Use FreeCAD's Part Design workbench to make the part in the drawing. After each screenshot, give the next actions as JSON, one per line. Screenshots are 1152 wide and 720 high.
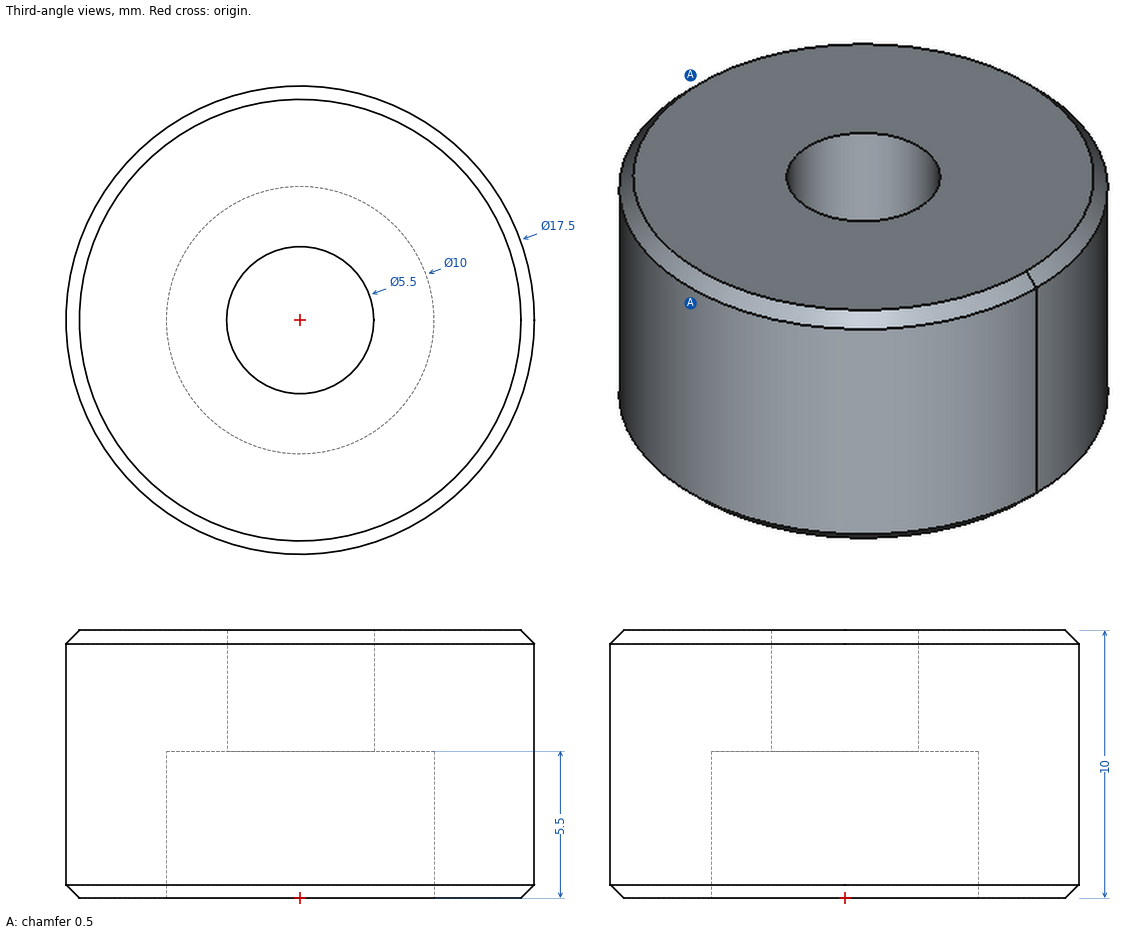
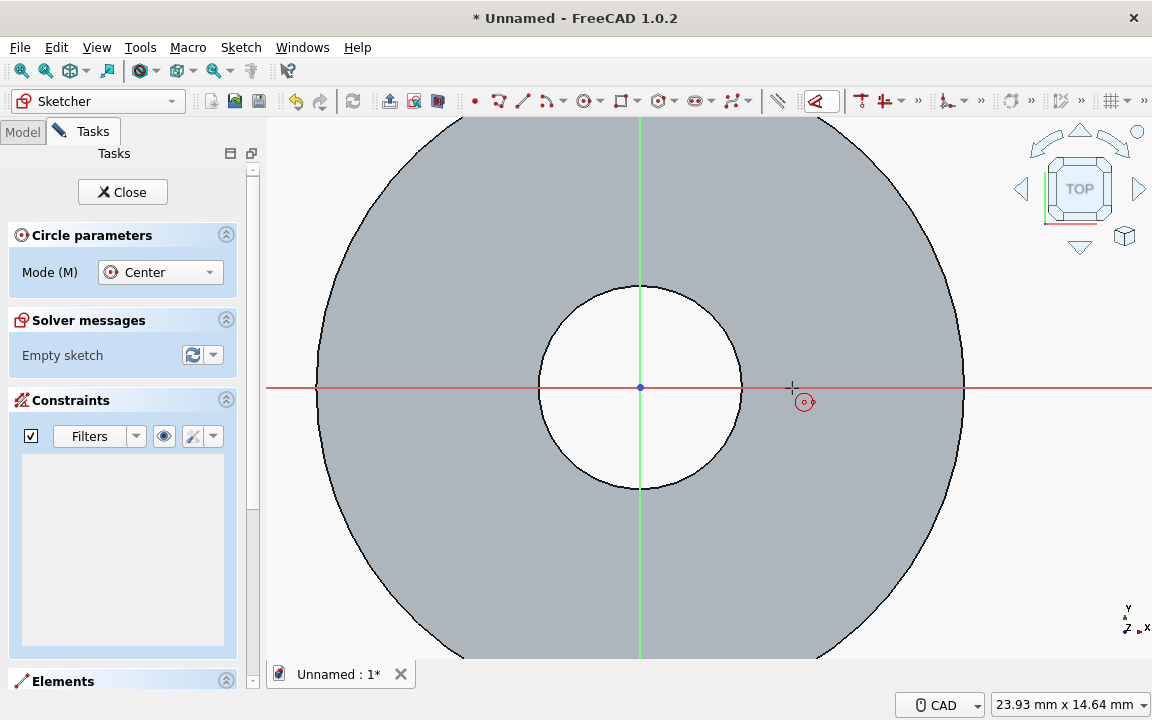
{"action": "left_click", "coordinate": [640, 388]}
{"action": "left_click", "coordinate": [771, 257]}
{"action": "key", "text": "Escape"}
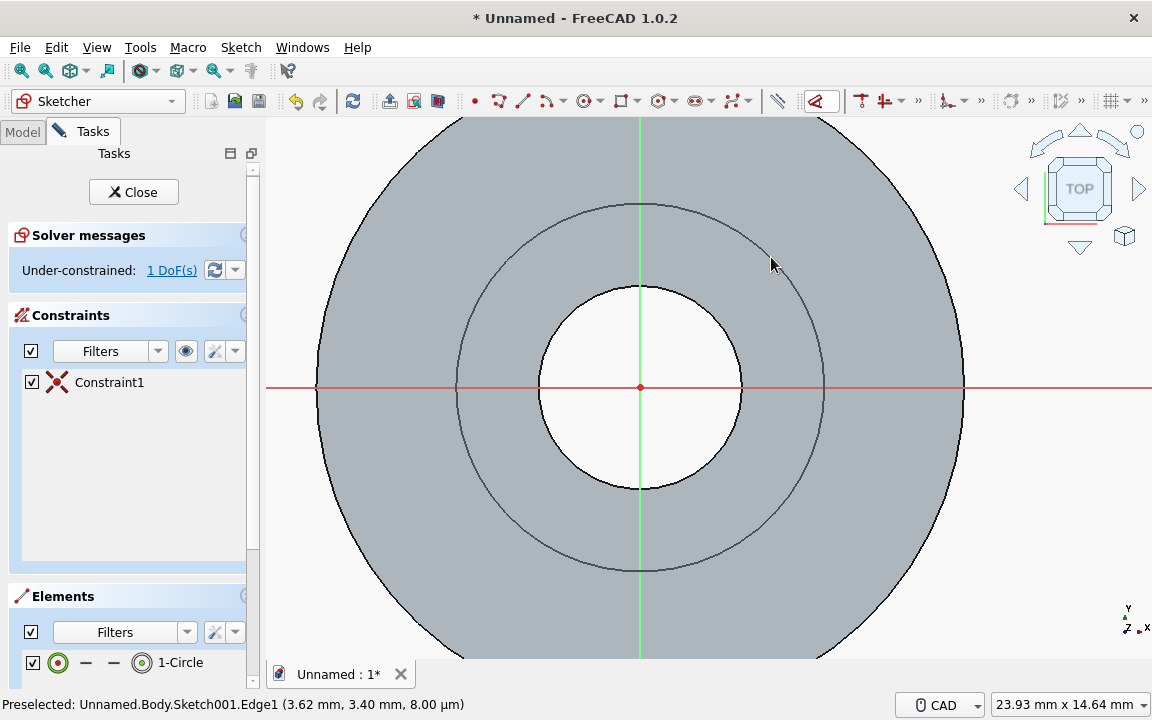
{"action": "left_click", "coordinate": [816, 102]}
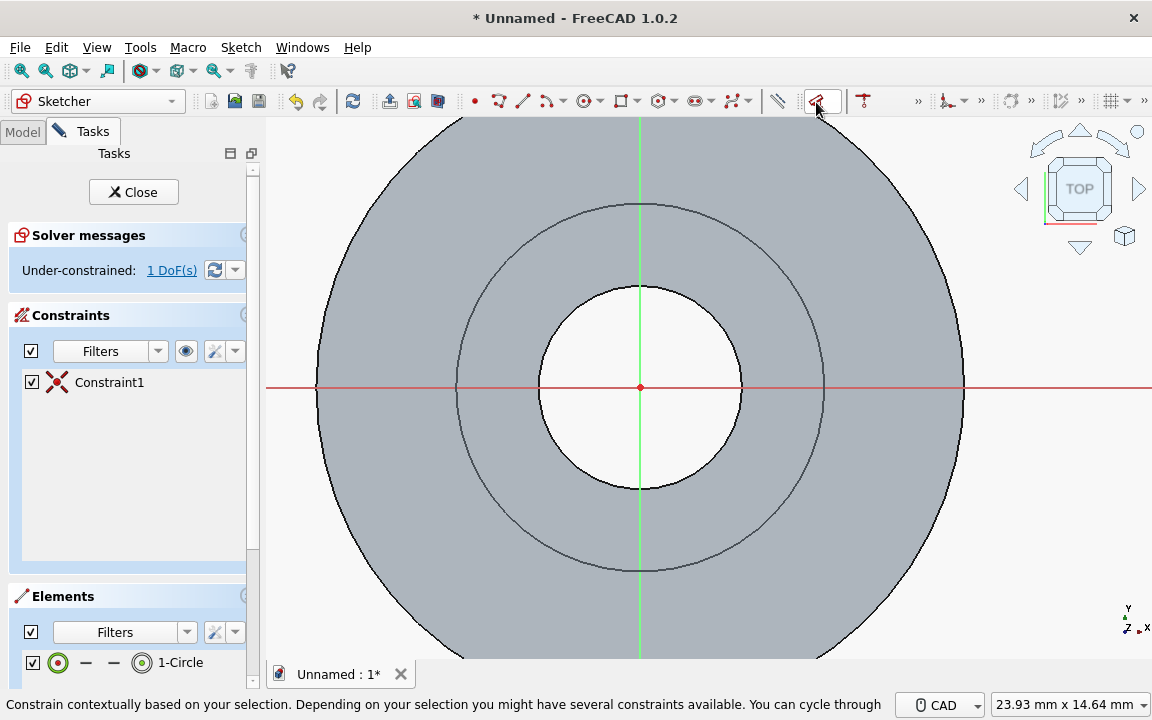
{"action": "left_click", "coordinate": [770, 257]}
{"action": "left_click", "coordinate": [793, 234]}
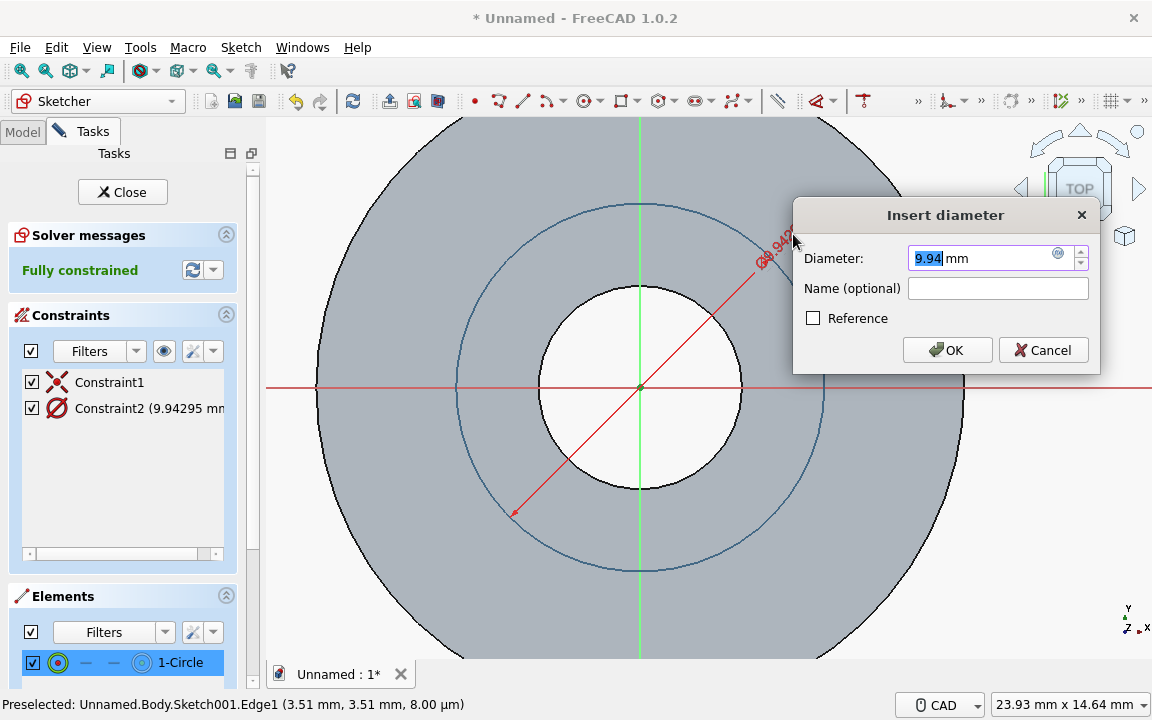
{"action": "type", "text": "10"}
{"action": "key", "text": "Return"}
{"action": "key", "text": "Escape"}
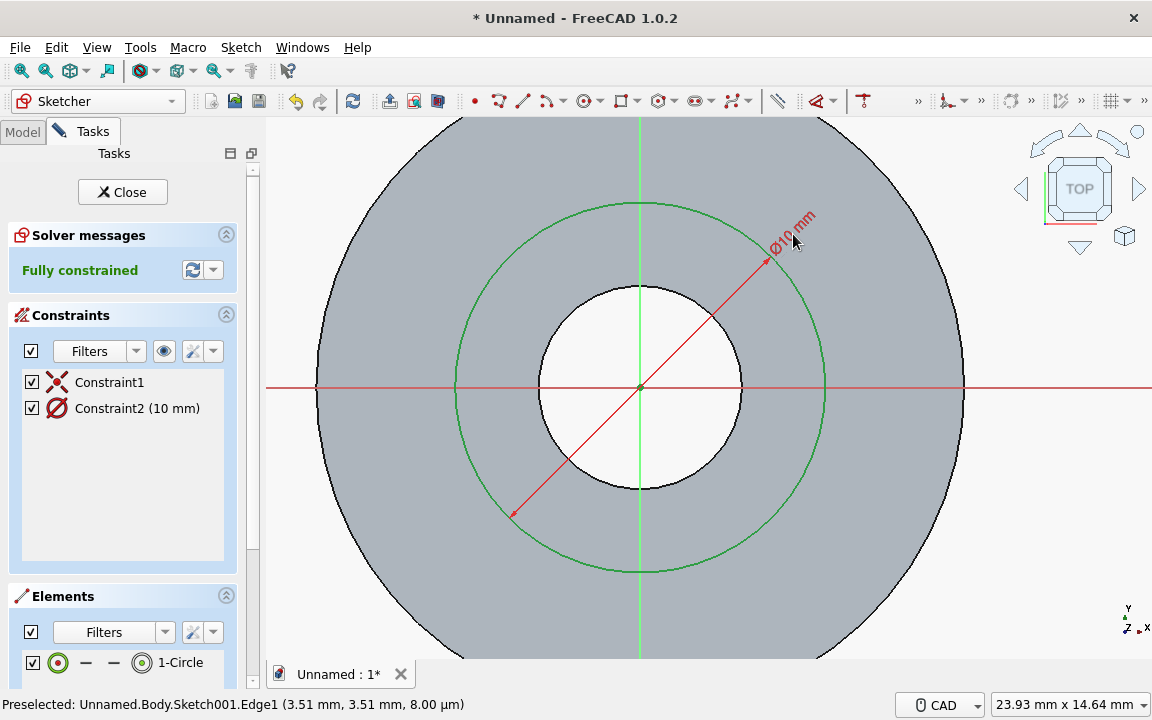
{"action": "left_click", "coordinate": [123, 192]}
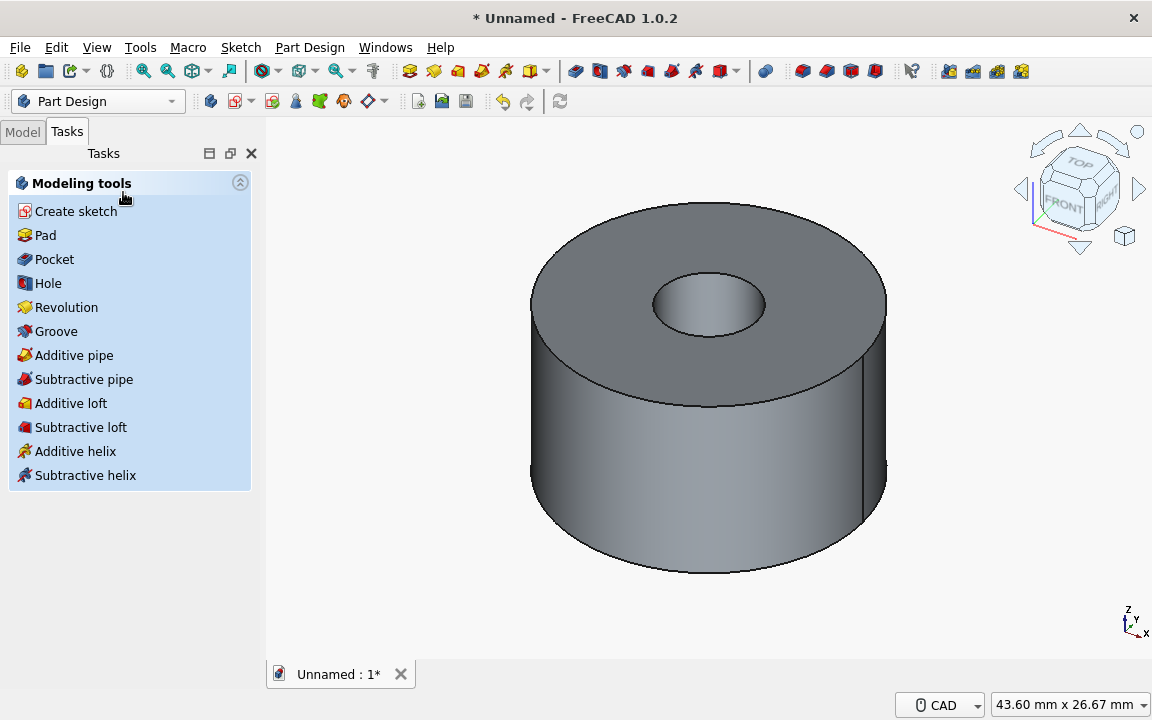
{"action": "left_click", "coordinate": [576, 72]}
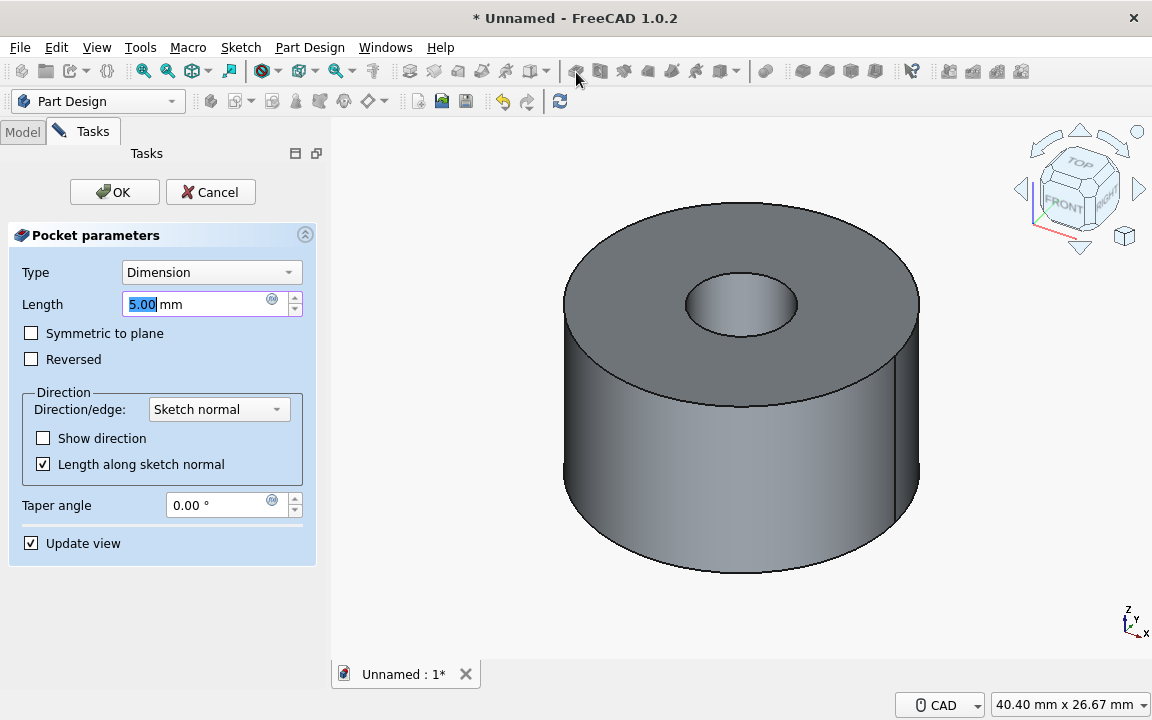
{"action": "type", "text": "5.5"}
{"action": "key", "text": "Tab"}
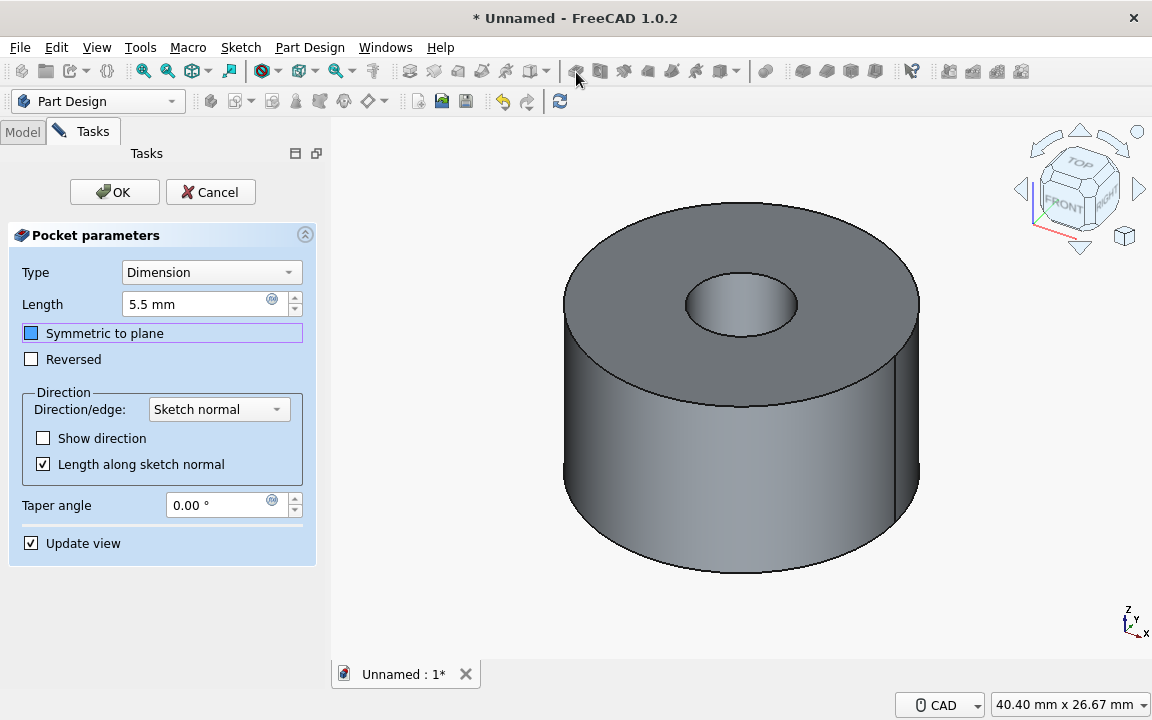
{"action": "left_click", "coordinate": [30, 359]}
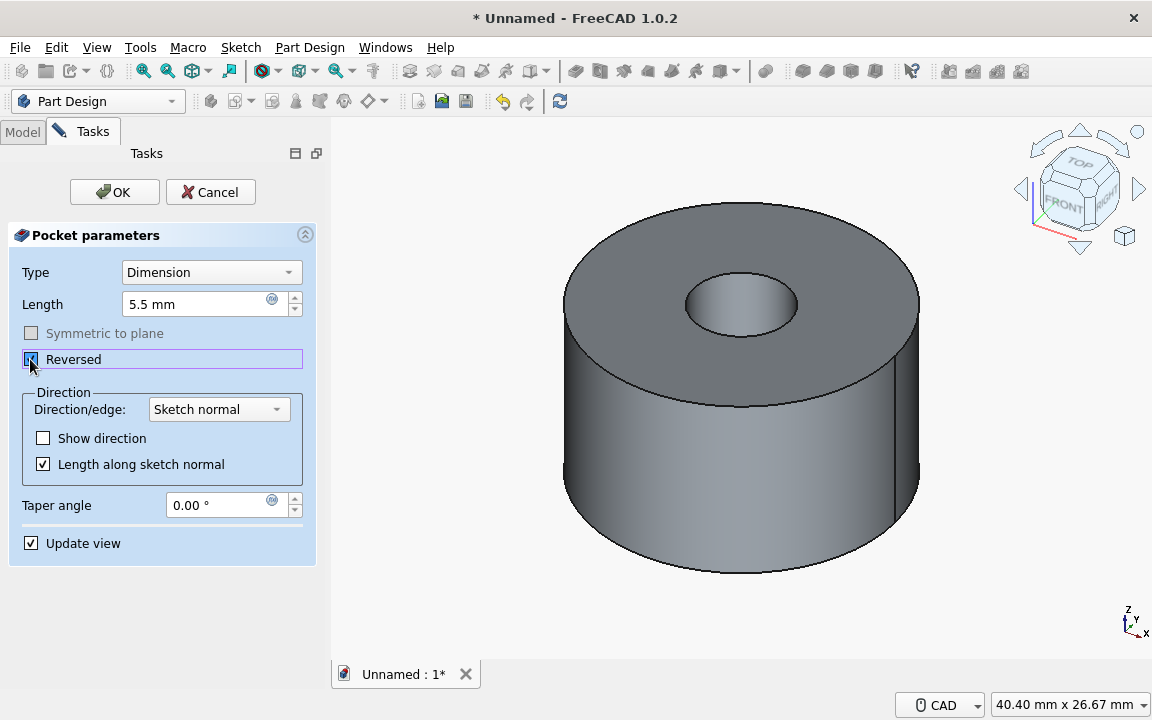
{"action": "left_click", "coordinate": [115, 192]}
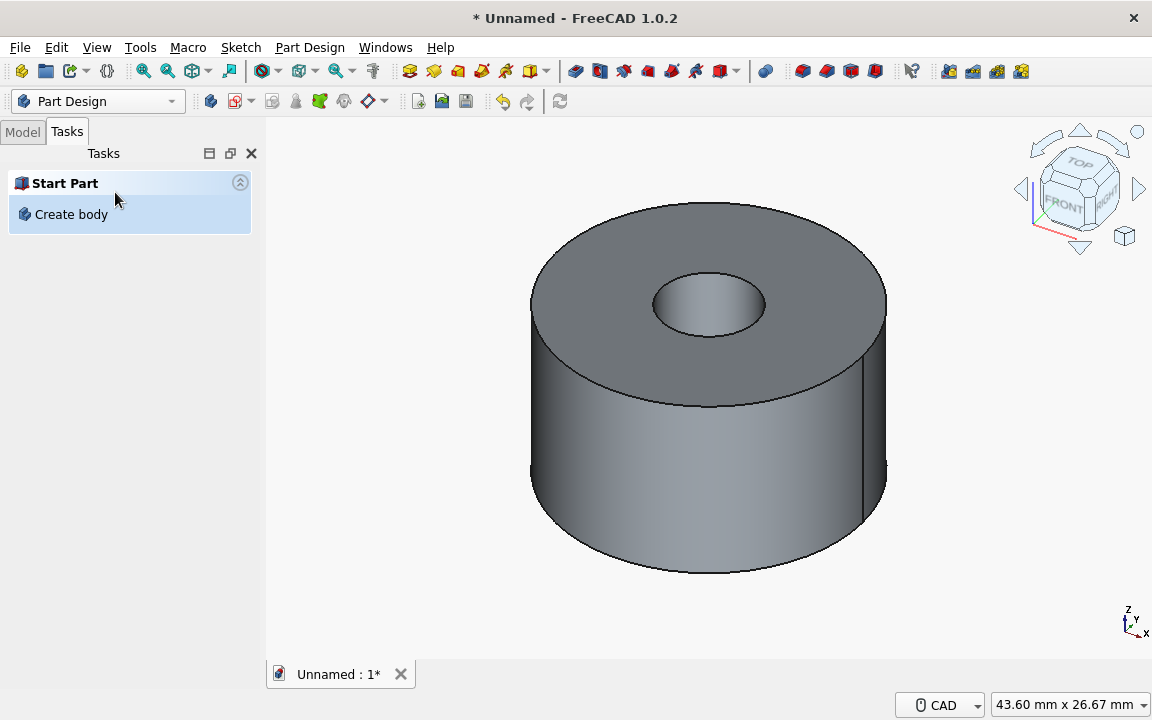
{"action": "left_click", "coordinate": [532, 314]}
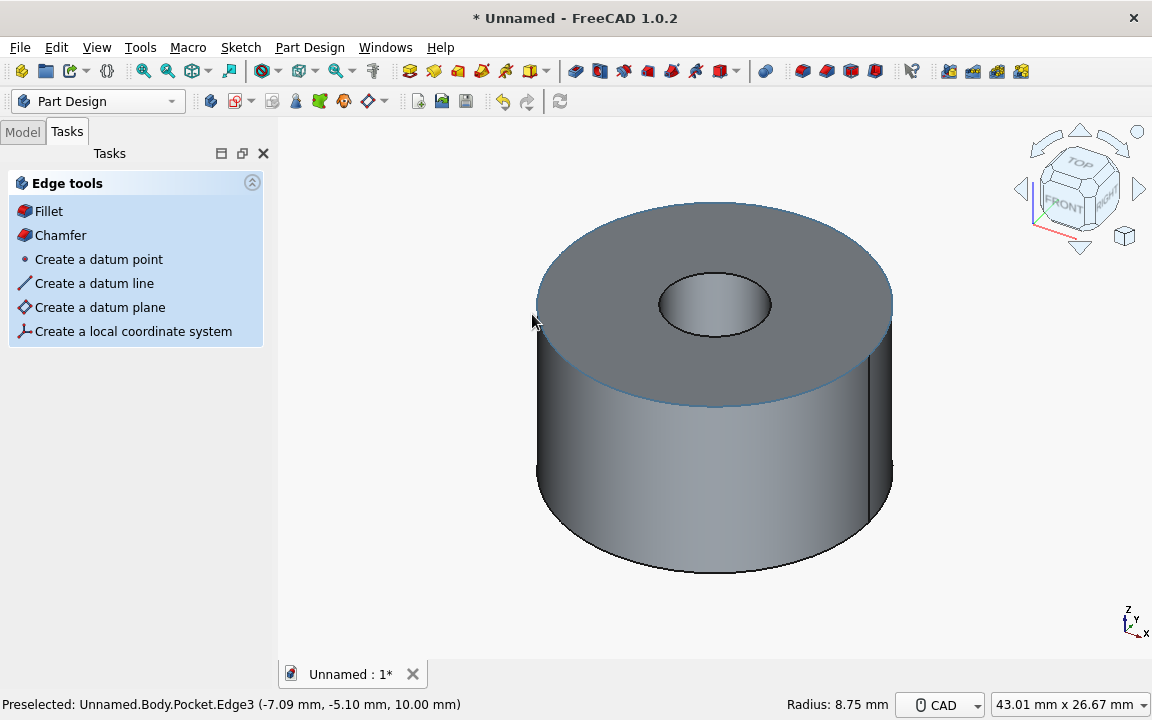
{"action": "key", "text": "0"}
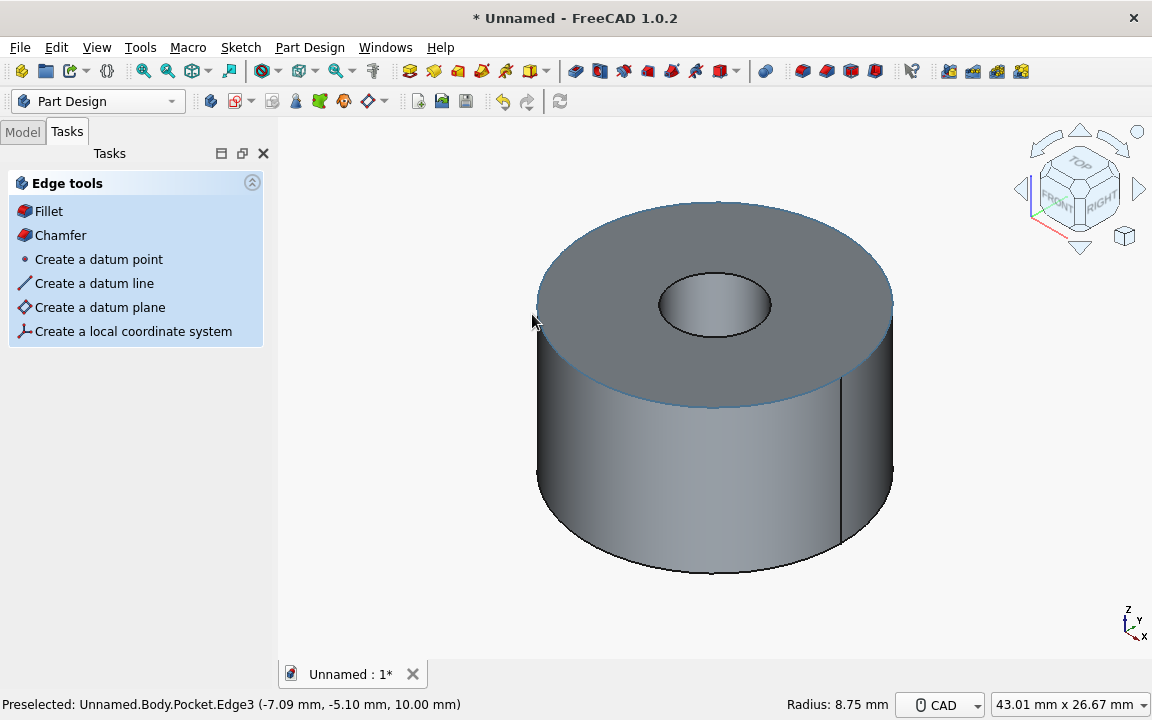
{"action": "key", "text": "2"}